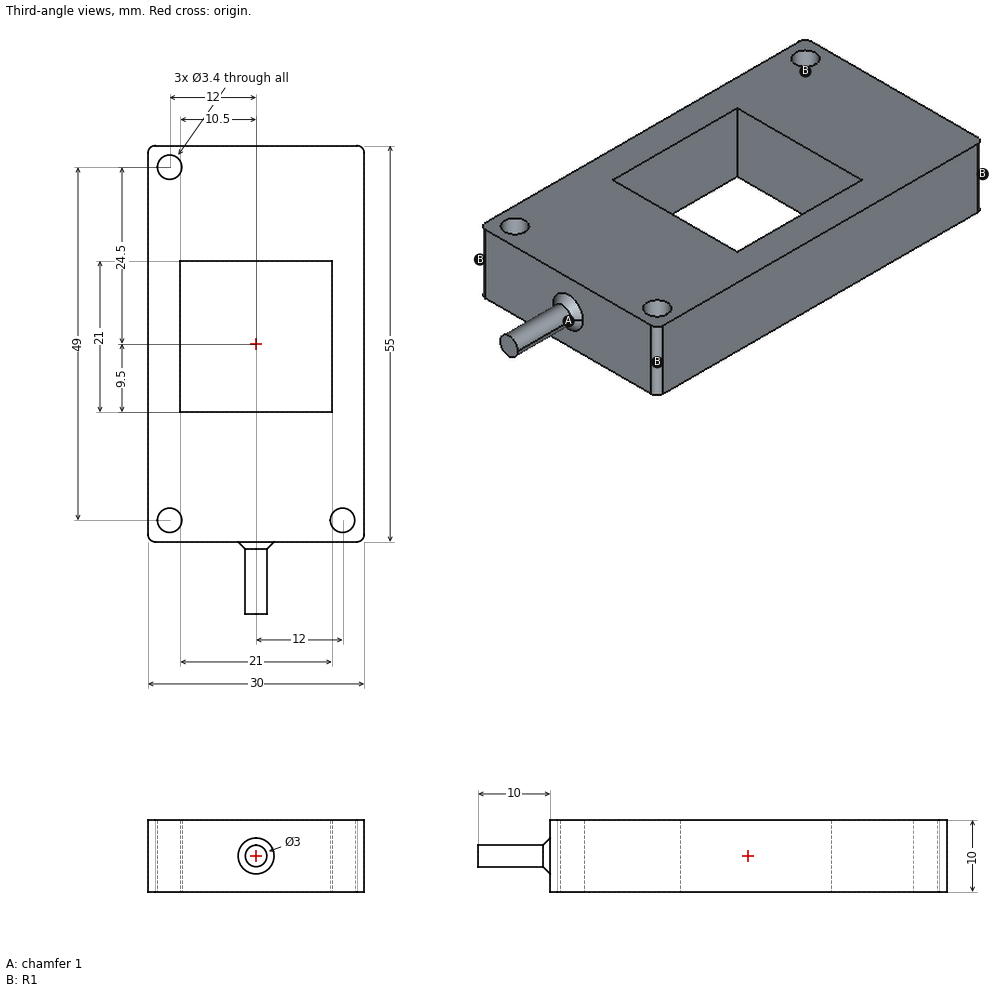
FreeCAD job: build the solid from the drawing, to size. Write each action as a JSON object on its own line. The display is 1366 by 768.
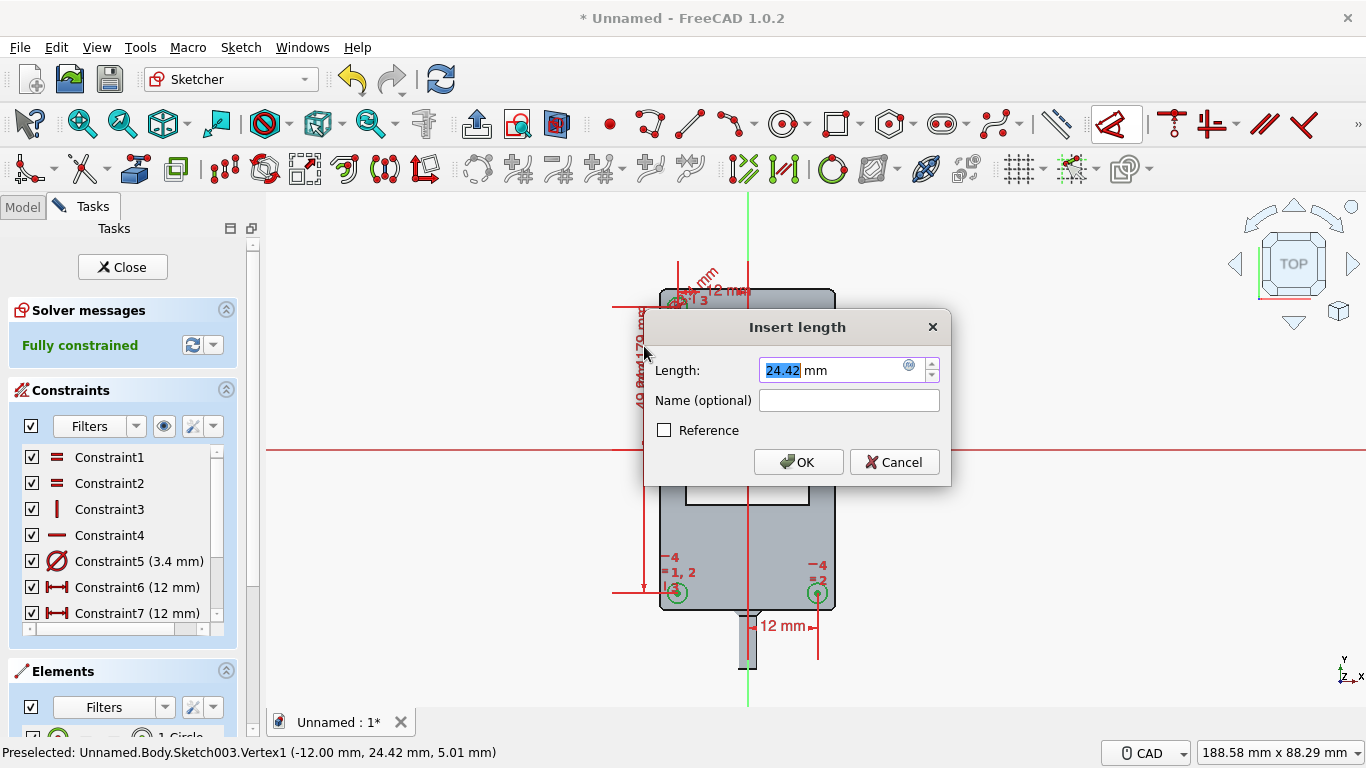
{"action": "type", "text": "24.5"}
{"action": "key", "text": "Return"}
{"action": "key", "text": "Escape"}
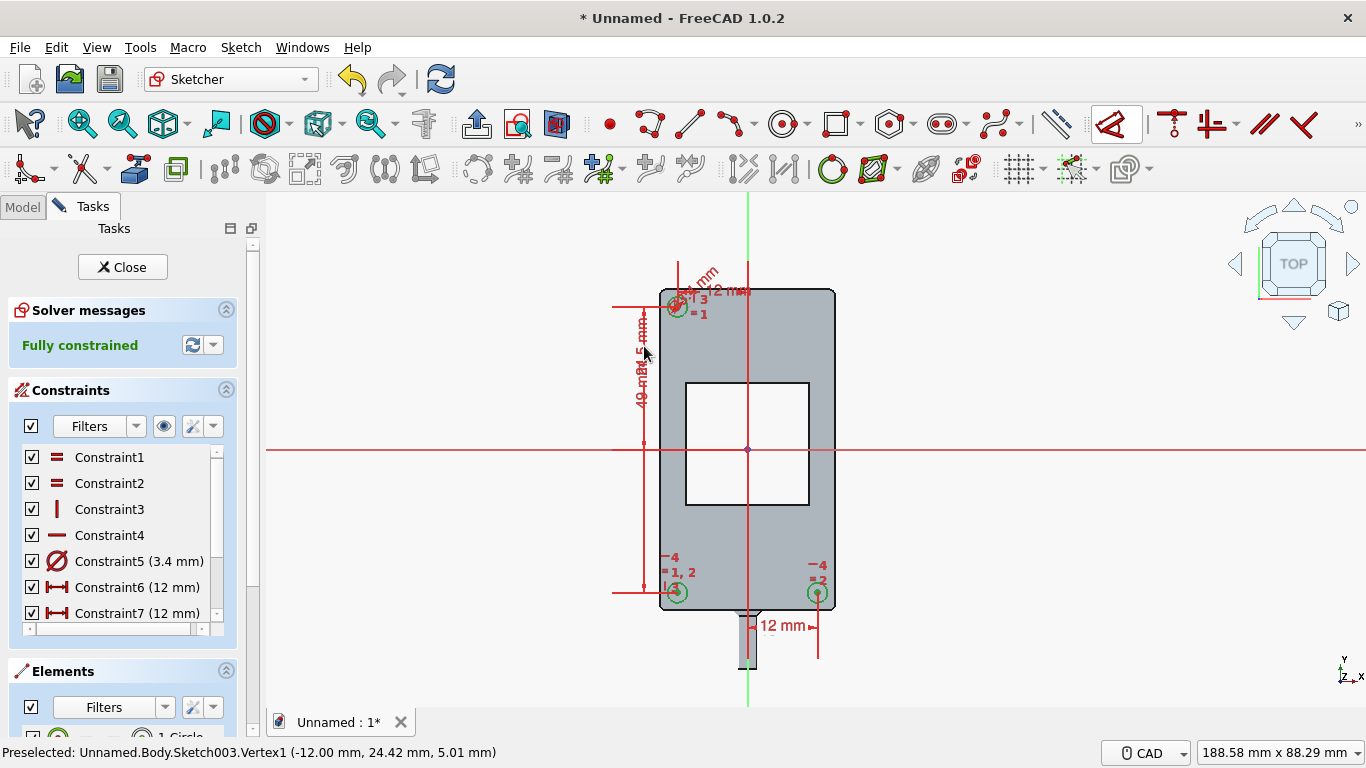
{"action": "left_click", "coordinate": [123, 267]}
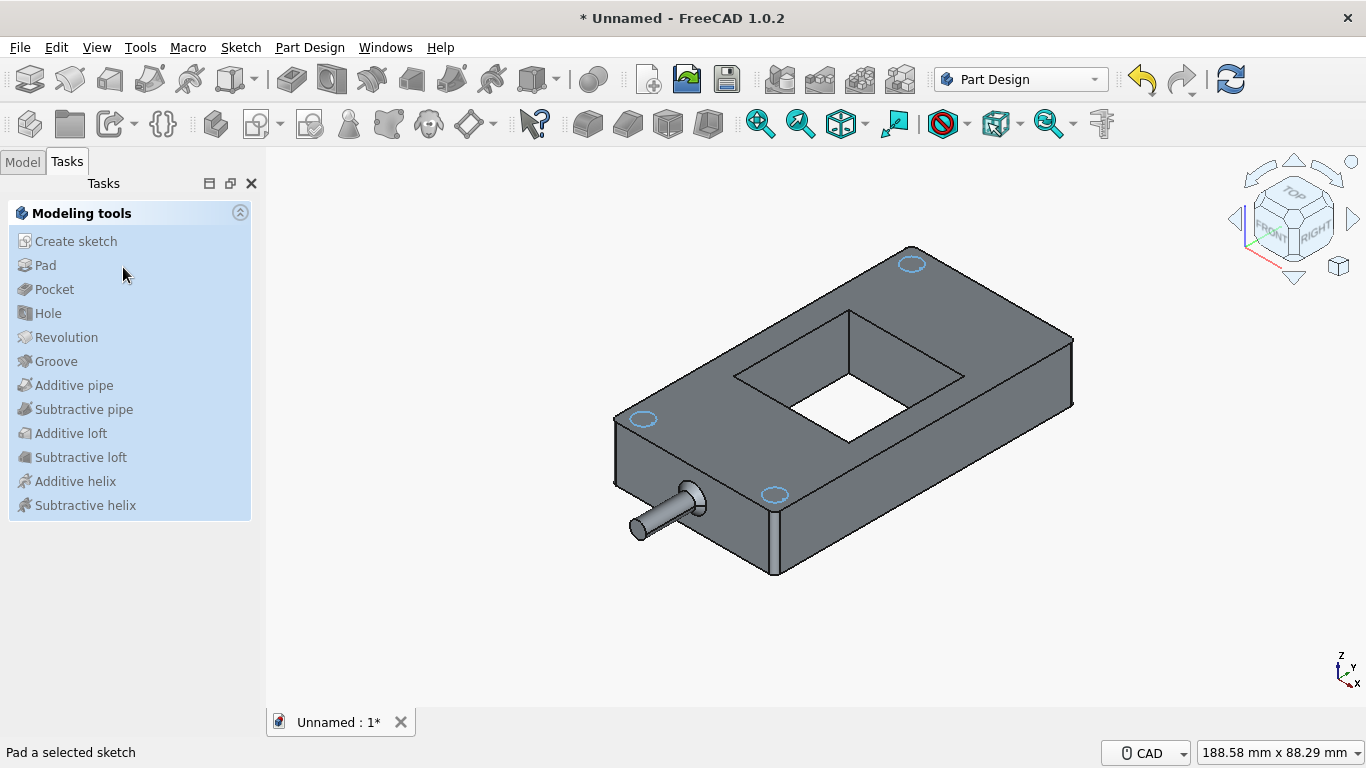
{"action": "left_click", "coordinate": [332, 80]}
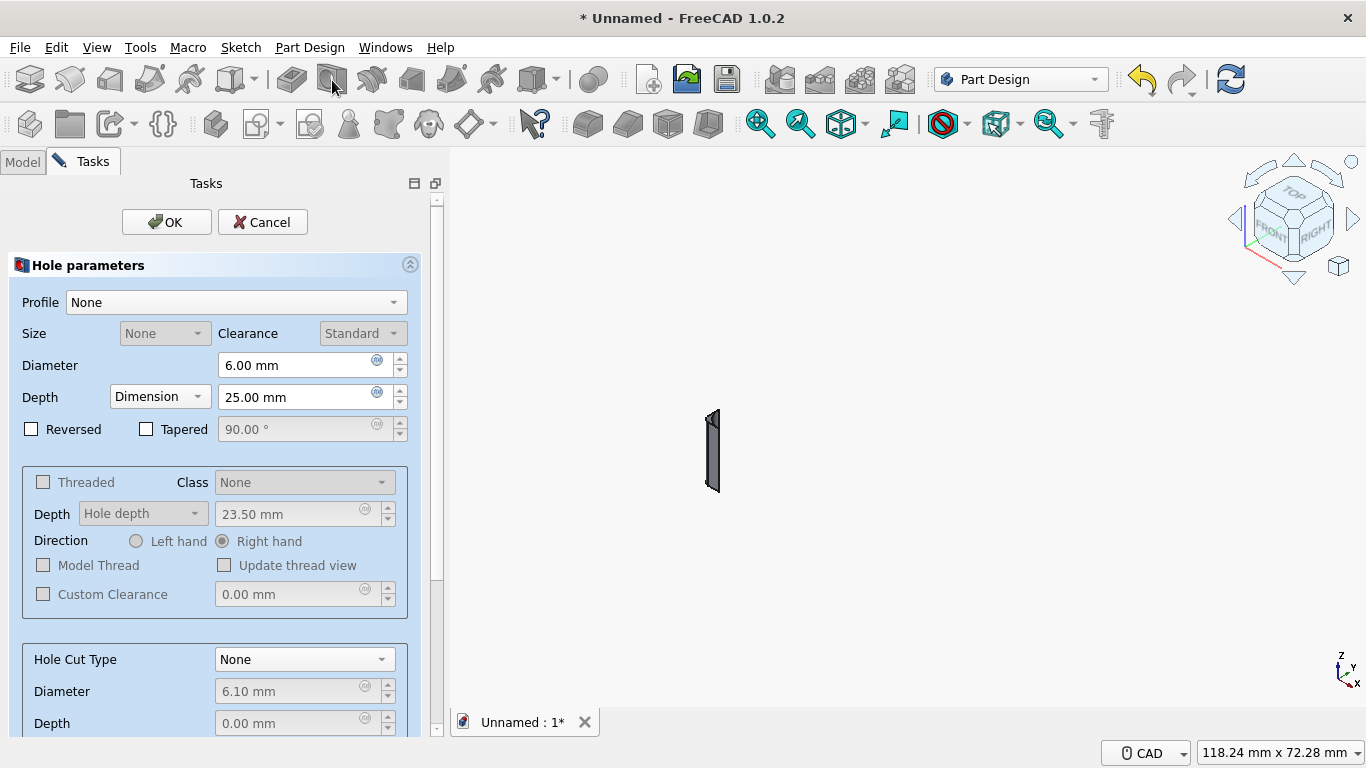
{"action": "triple_click", "coordinate": [305, 365]}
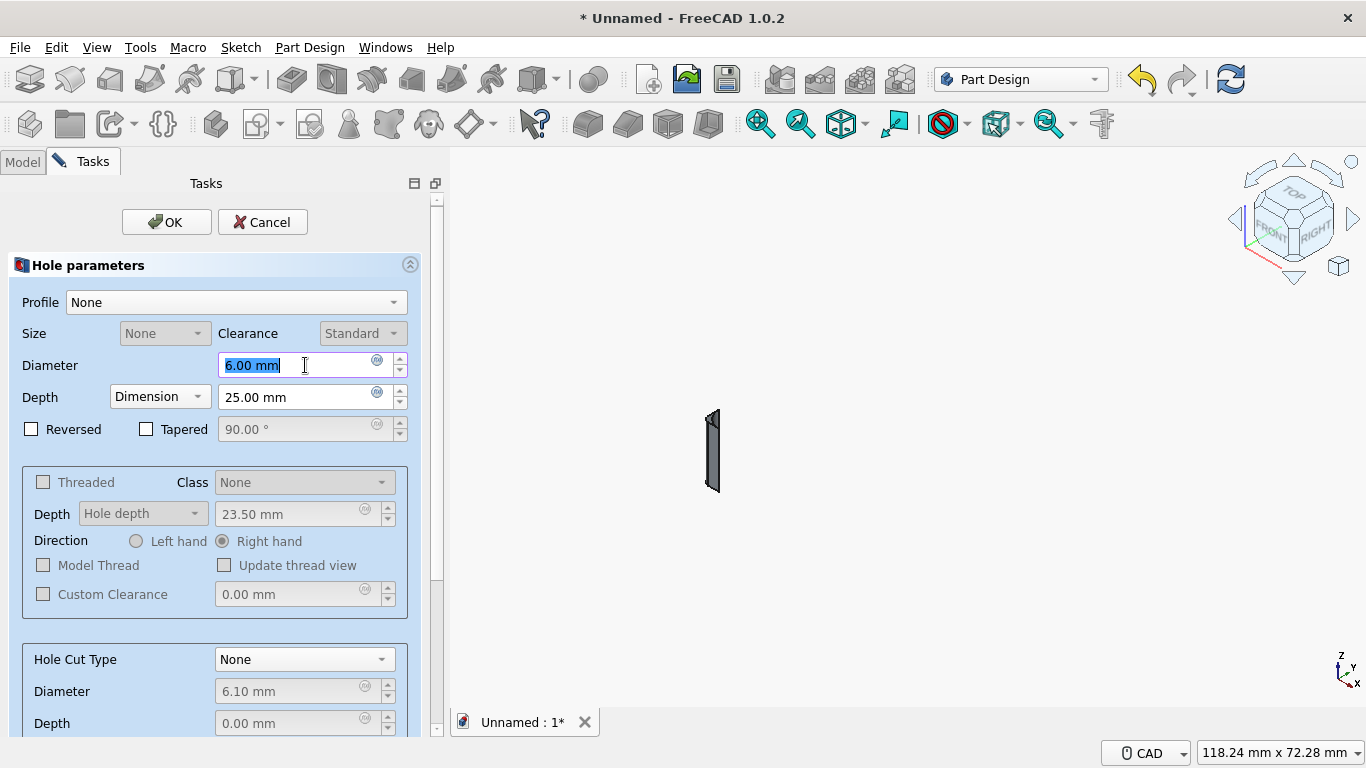
{"action": "type", "text": "3.4"}
{"action": "key", "text": "Tab"}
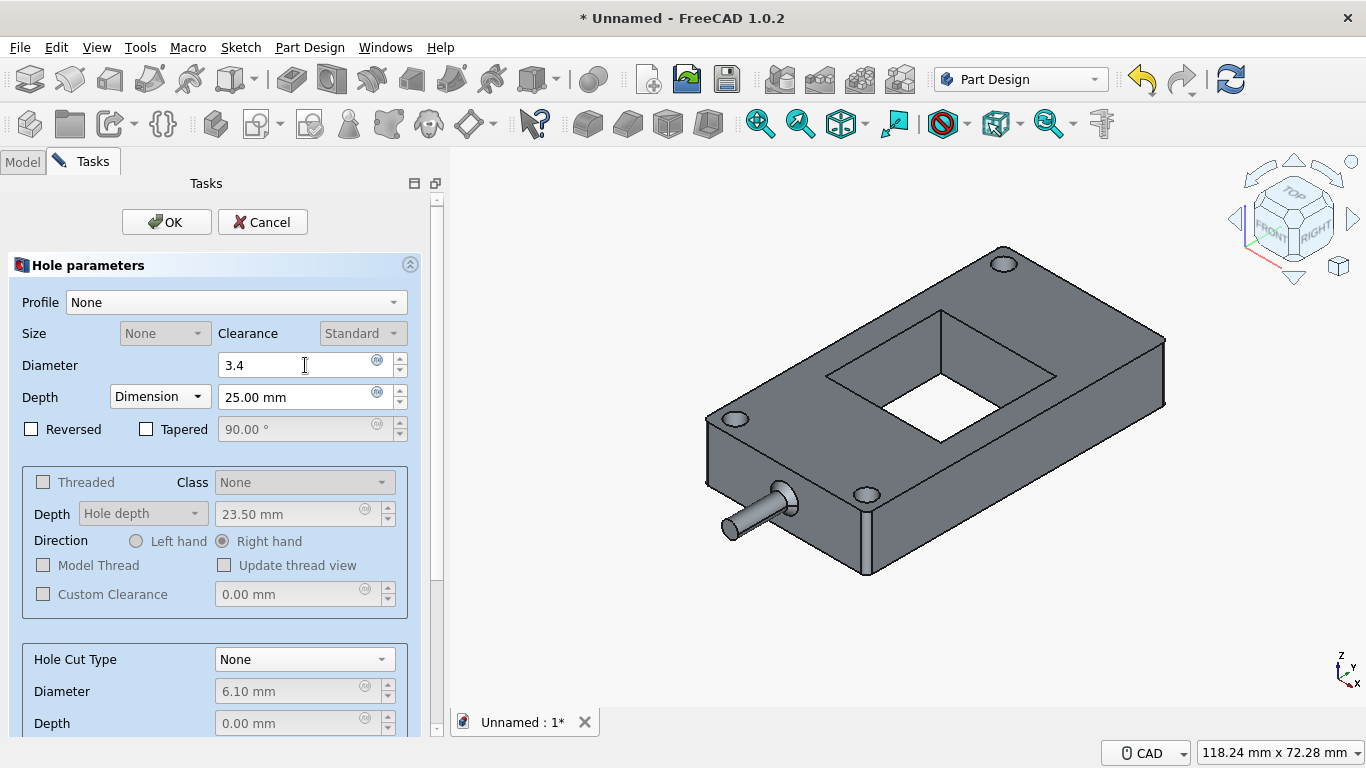
{"action": "left_click", "coordinate": [161, 396]}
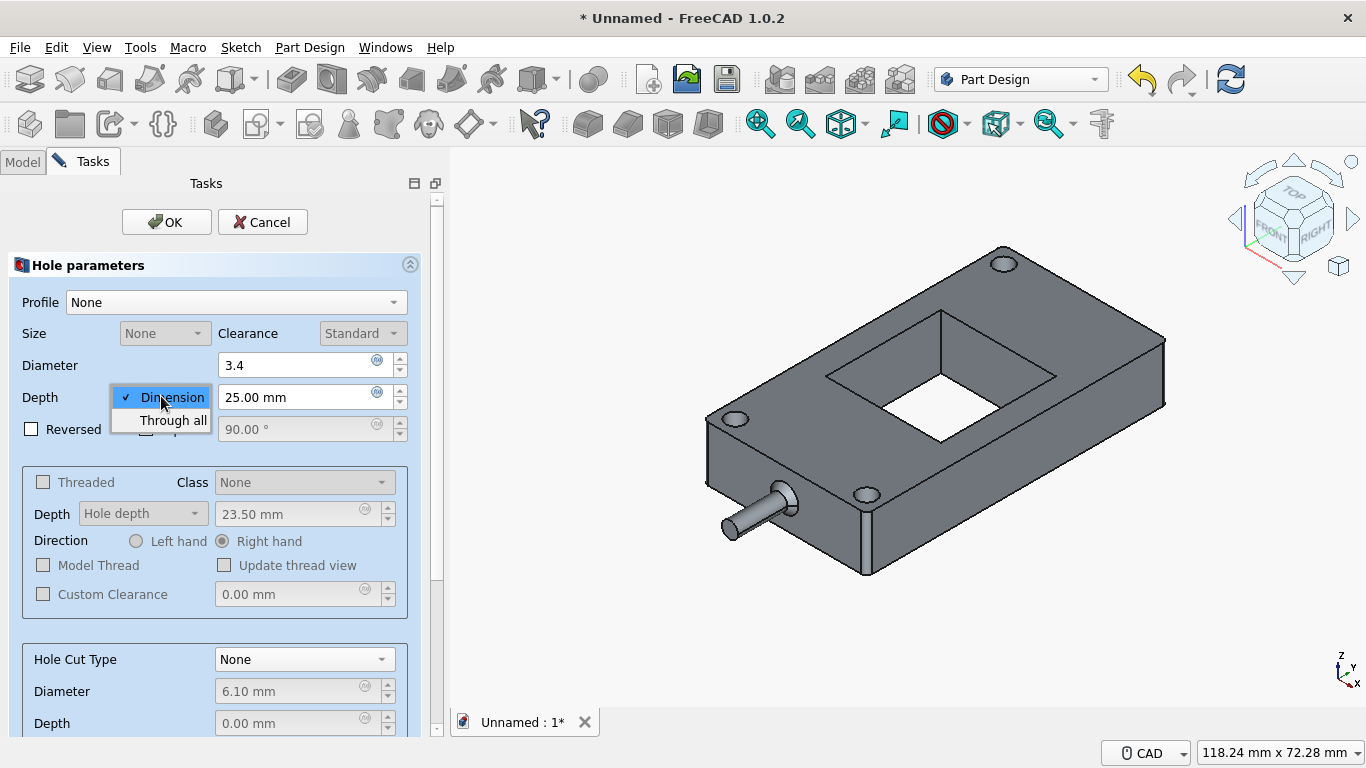
{"action": "left_click", "coordinate": [160, 420]}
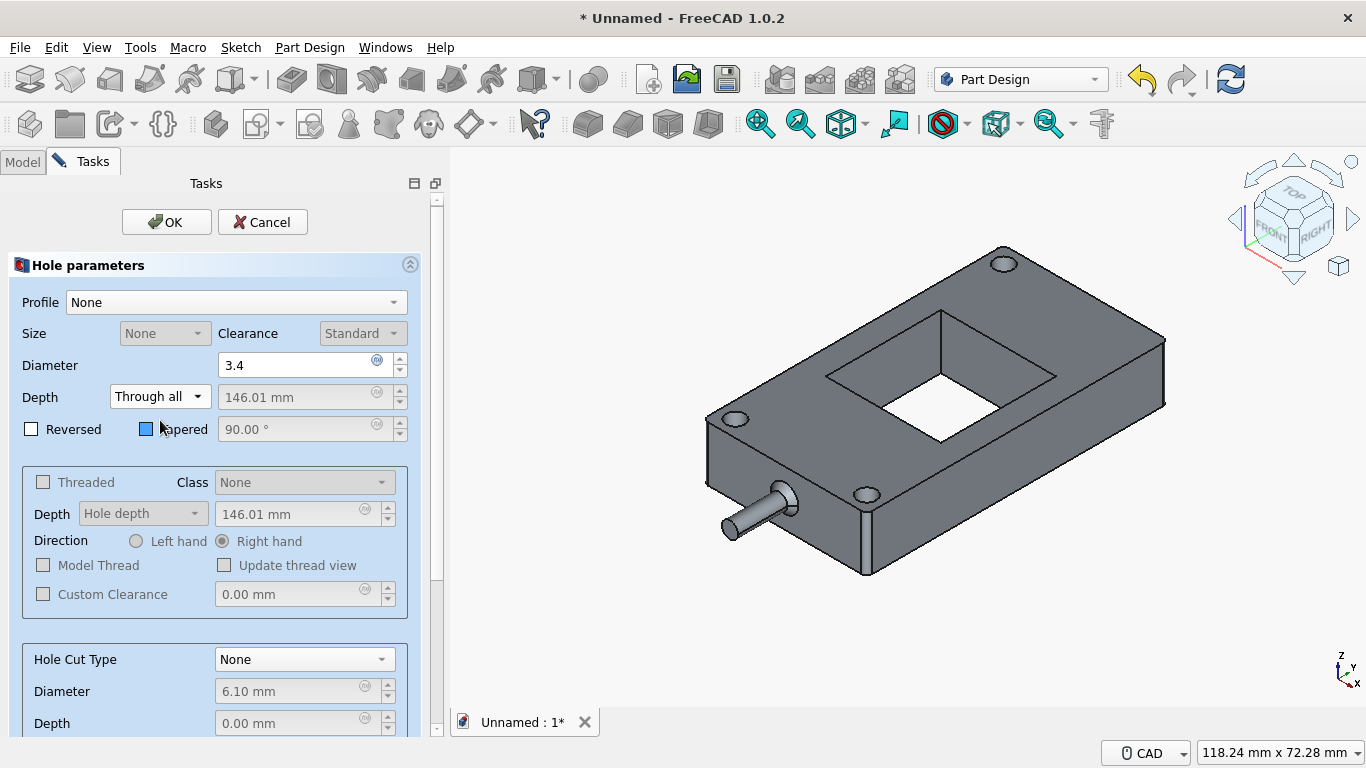
{"action": "left_click", "coordinate": [167, 222]}